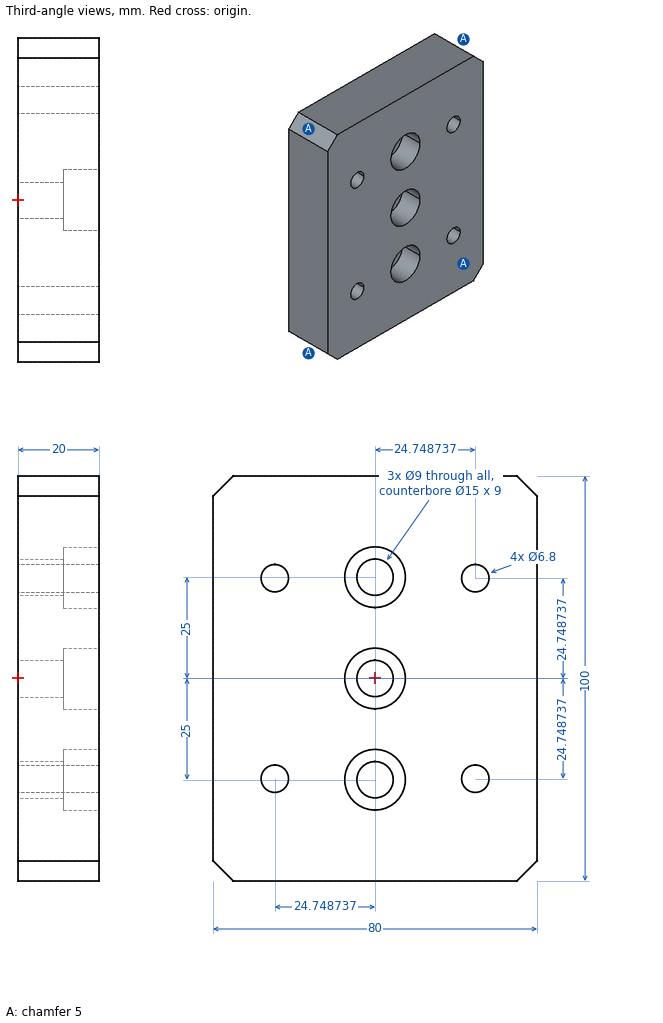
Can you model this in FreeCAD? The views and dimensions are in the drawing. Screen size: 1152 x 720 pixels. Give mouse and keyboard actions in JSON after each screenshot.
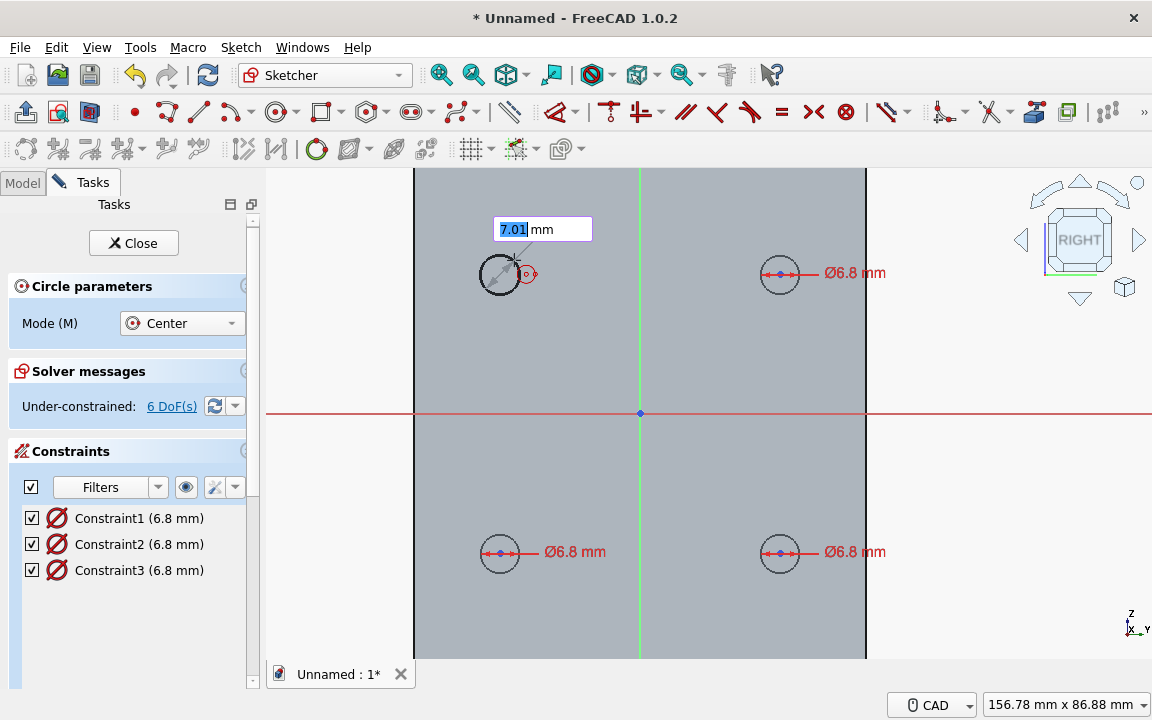
{"action": "type", "text": "6.8"}
{"action": "key", "text": "Return"}
{"action": "key", "text": "Escape"}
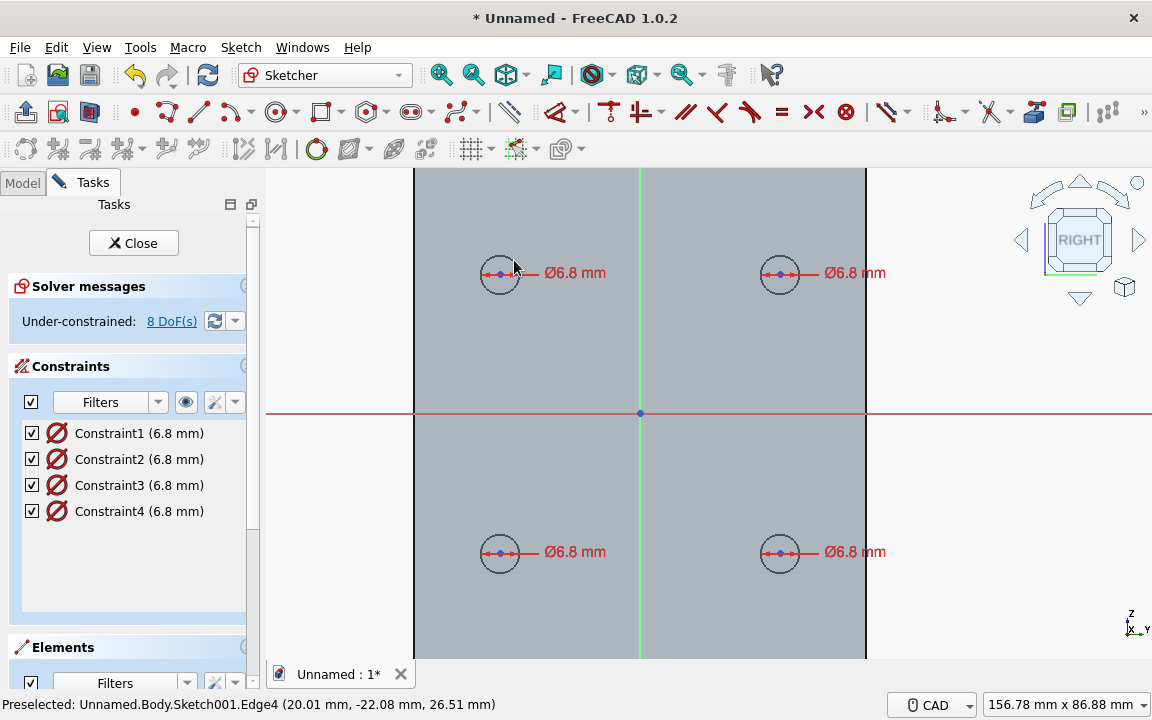
{"action": "left_click", "coordinate": [780, 275]}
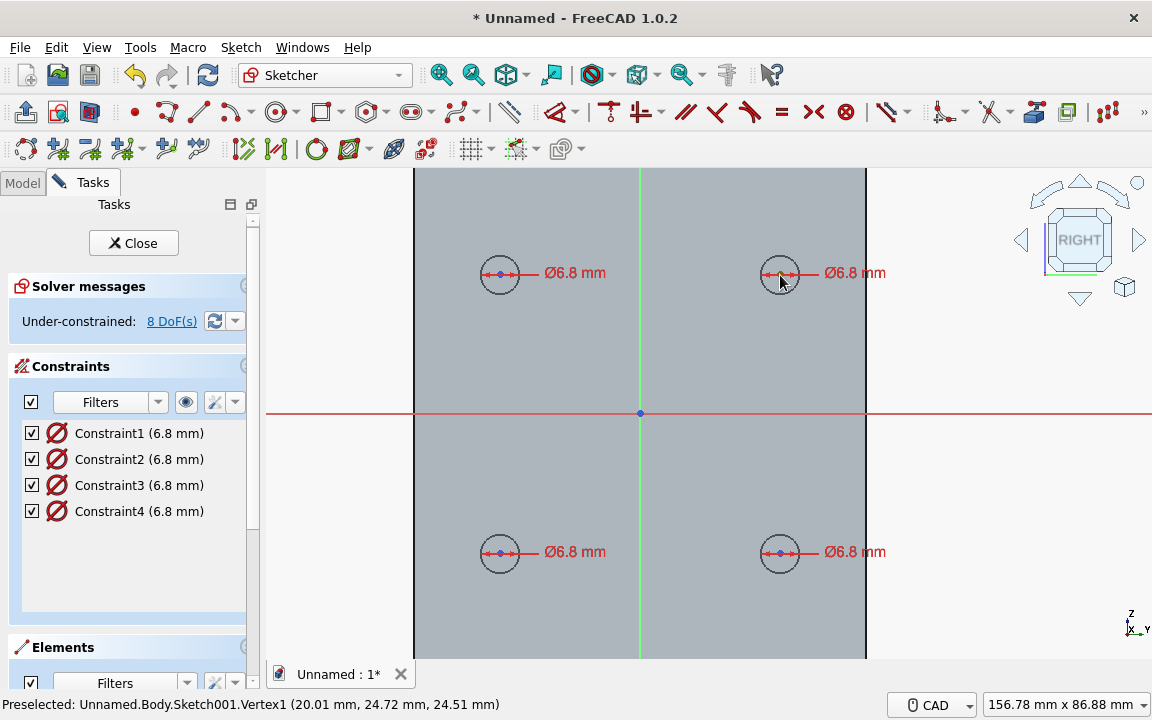
{"action": "left_click", "coordinate": [780, 554]}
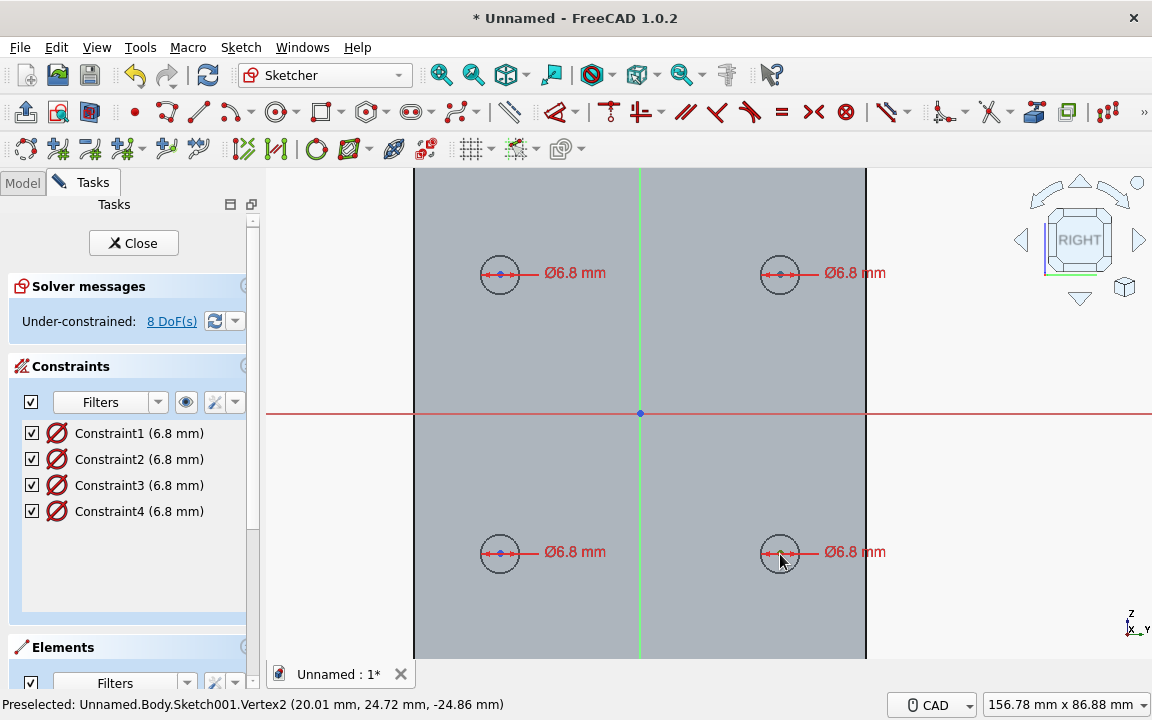
{"action": "key", "text": "v"}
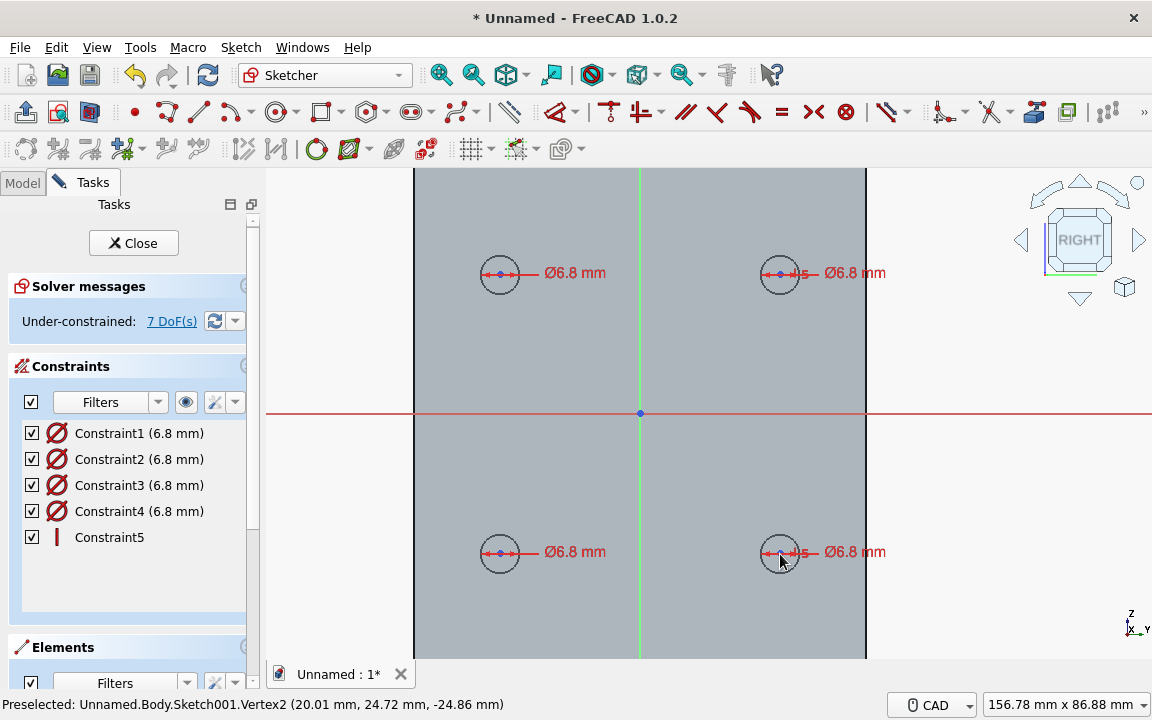
{"action": "left_click", "coordinate": [780, 554]}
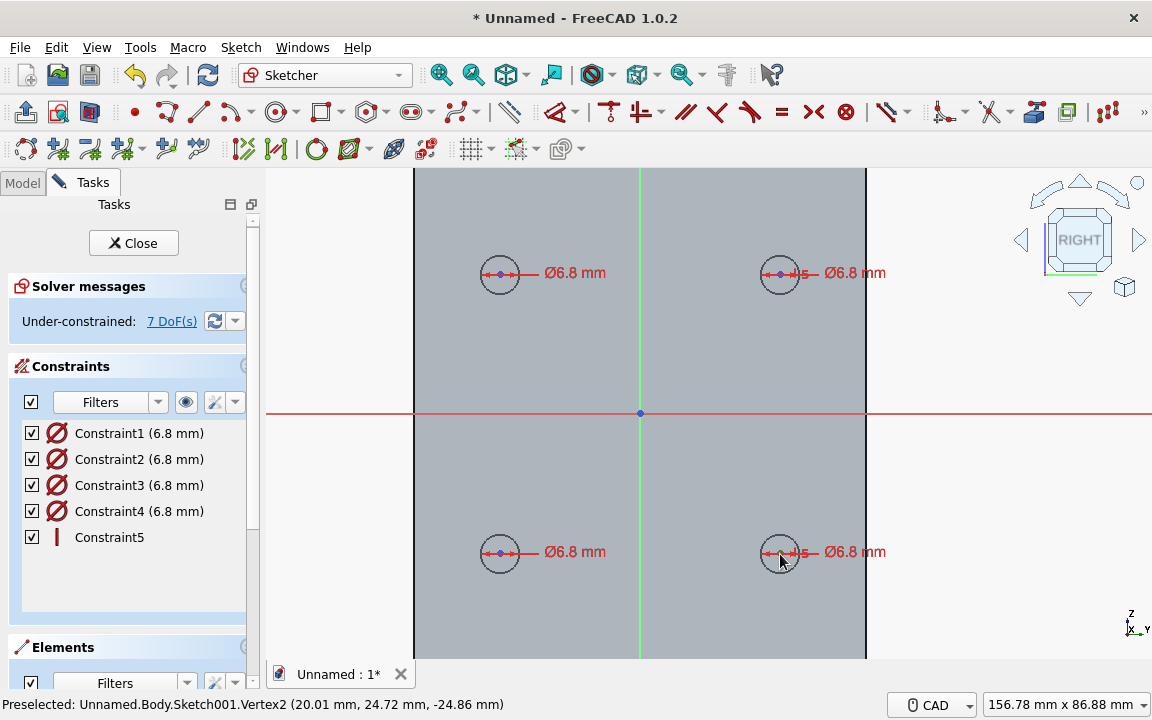
{"action": "left_click", "coordinate": [500, 554]}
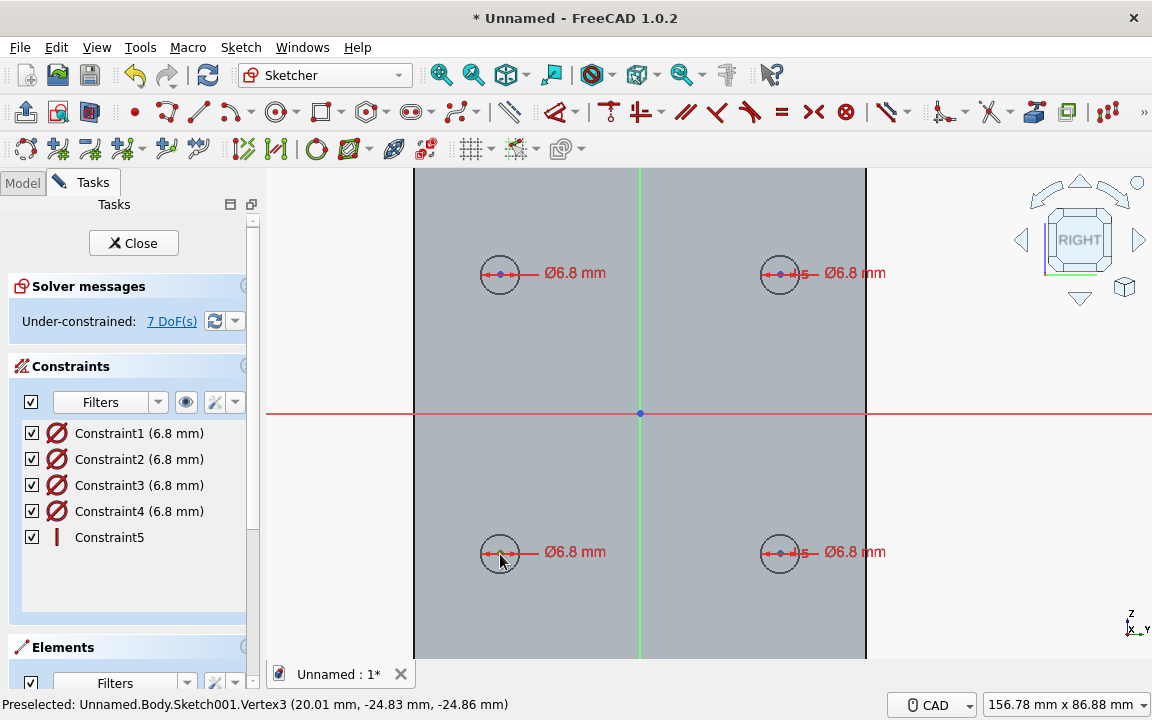
{"action": "key", "text": "h"}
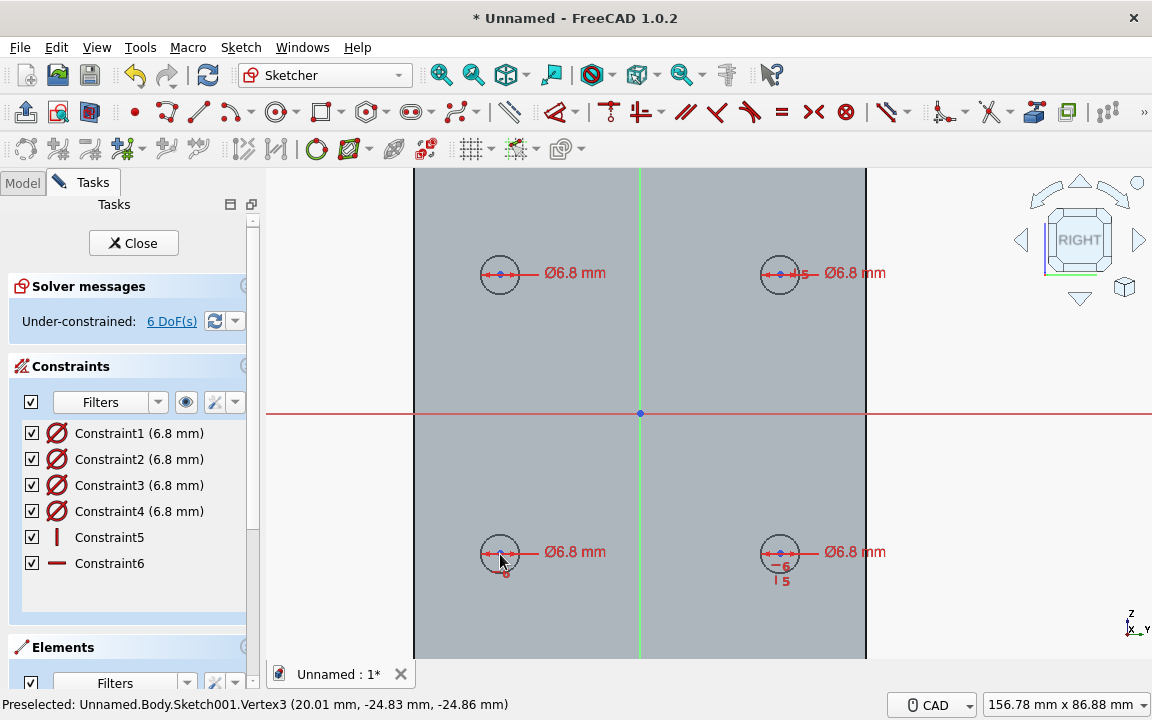
{"action": "left_click", "coordinate": [500, 554]}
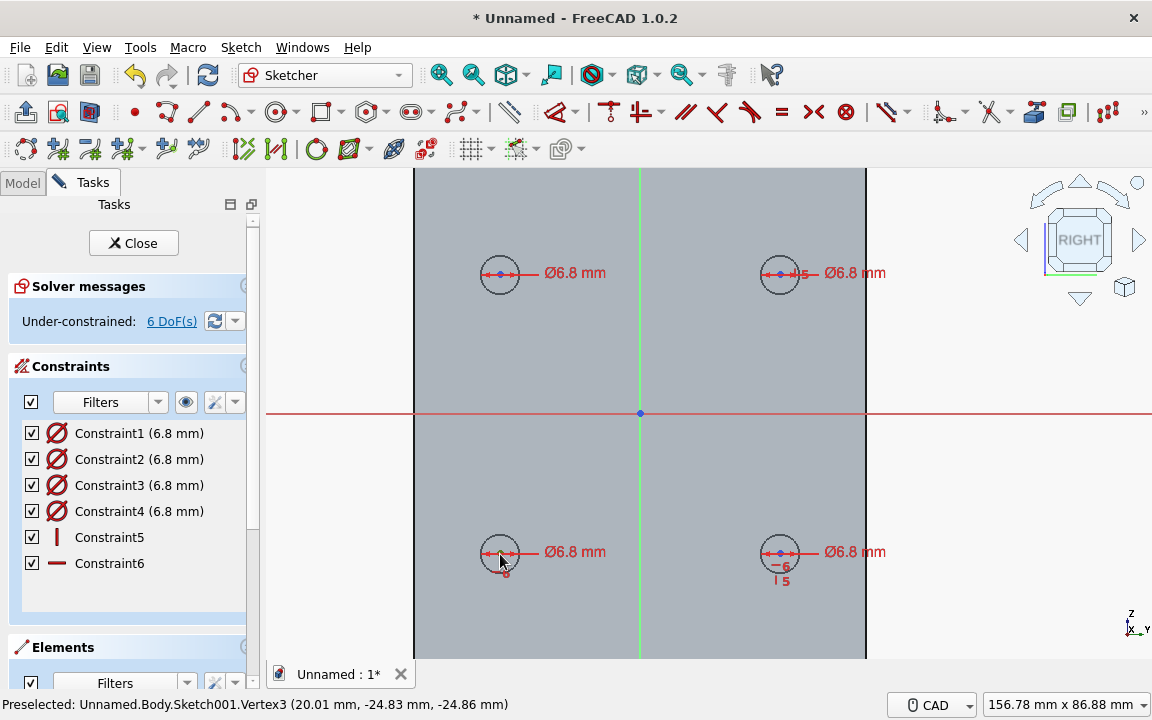
{"action": "left_click", "coordinate": [500, 275]}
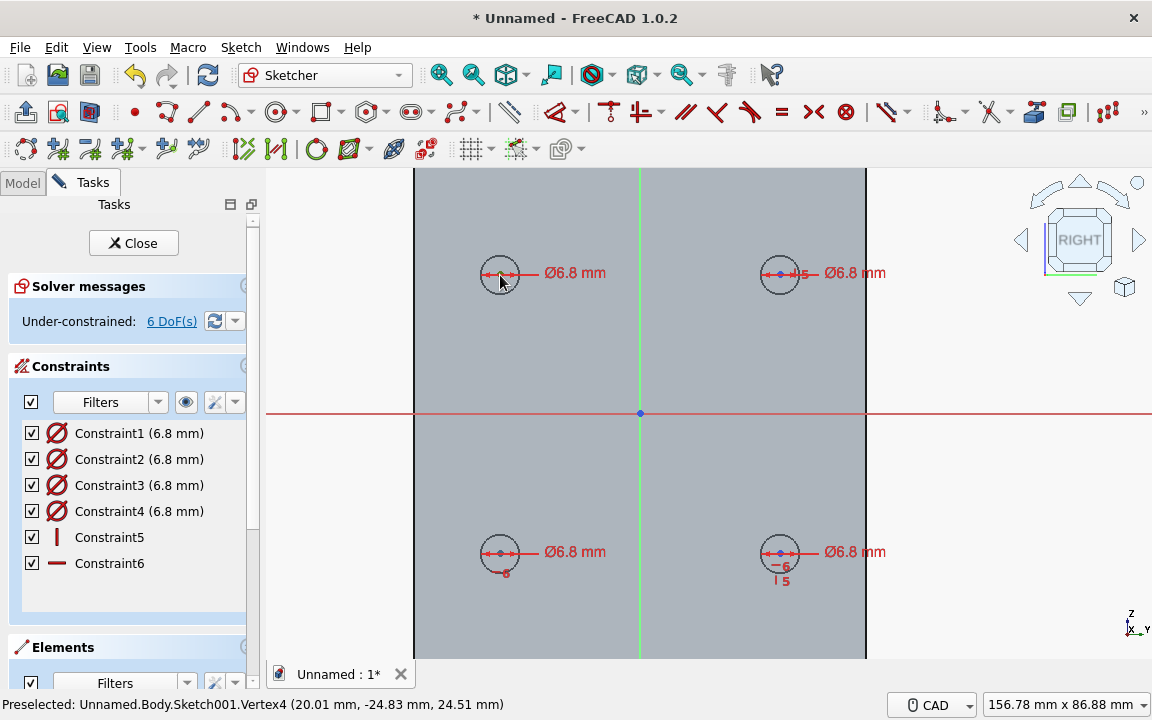
{"action": "key", "text": "v"}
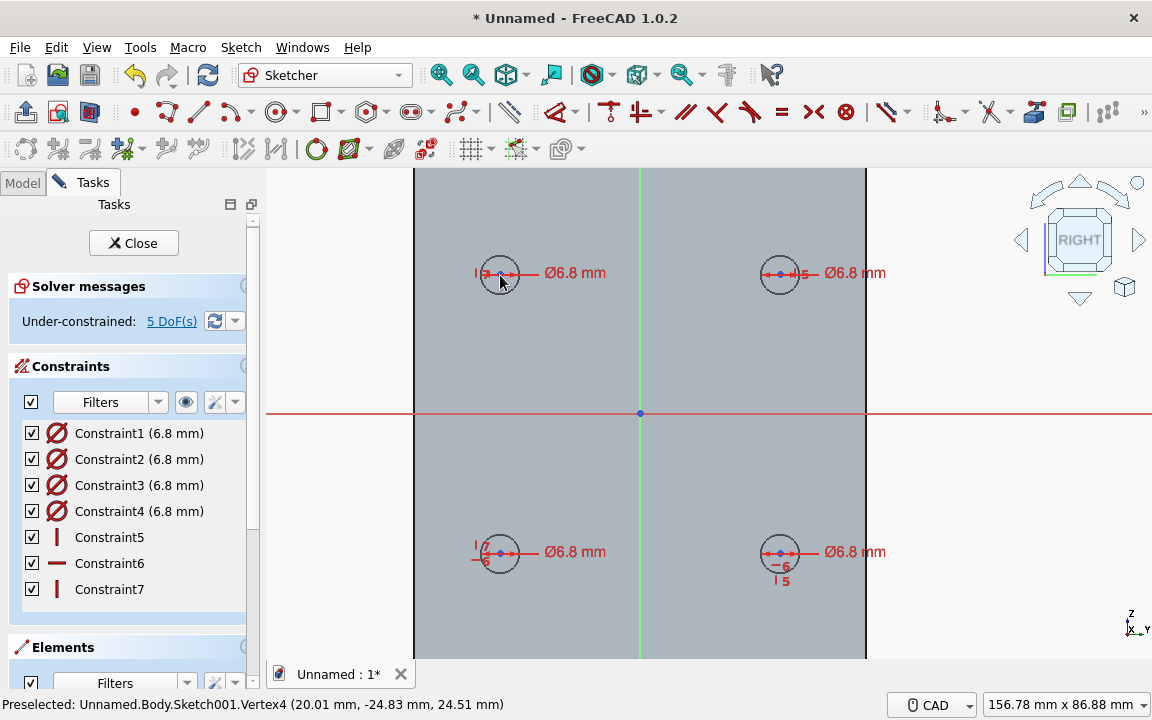
{"action": "left_click", "coordinate": [780, 275]}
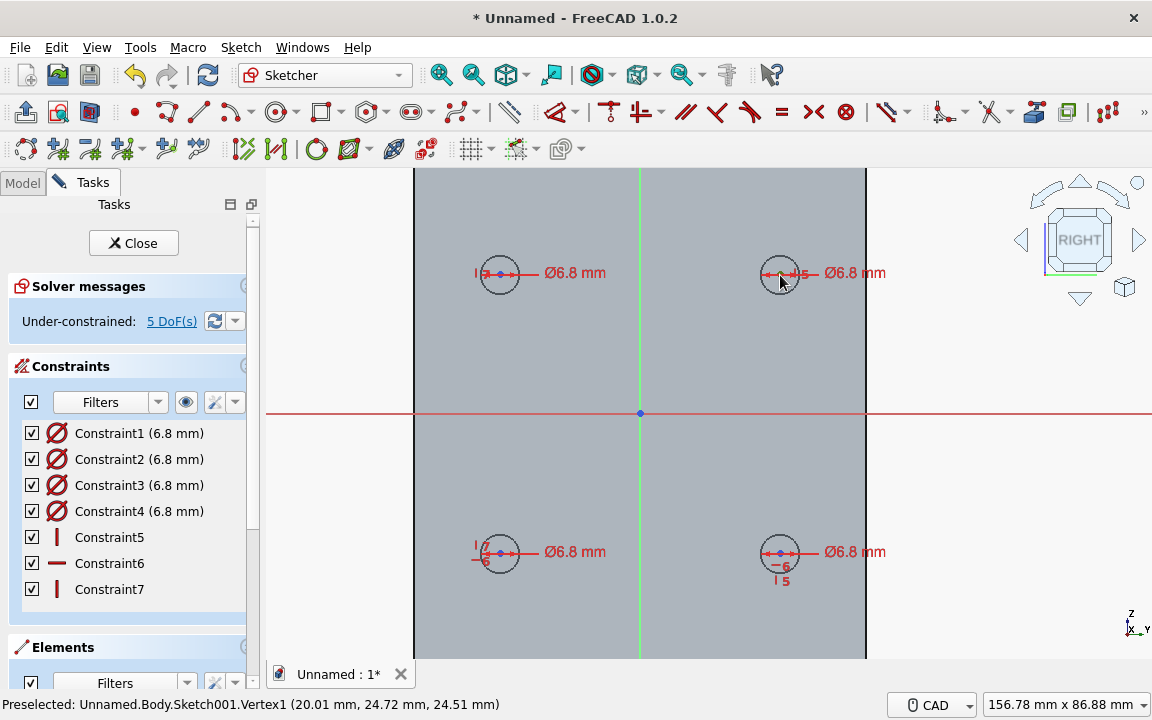
{"action": "left_click", "coordinate": [500, 275]}